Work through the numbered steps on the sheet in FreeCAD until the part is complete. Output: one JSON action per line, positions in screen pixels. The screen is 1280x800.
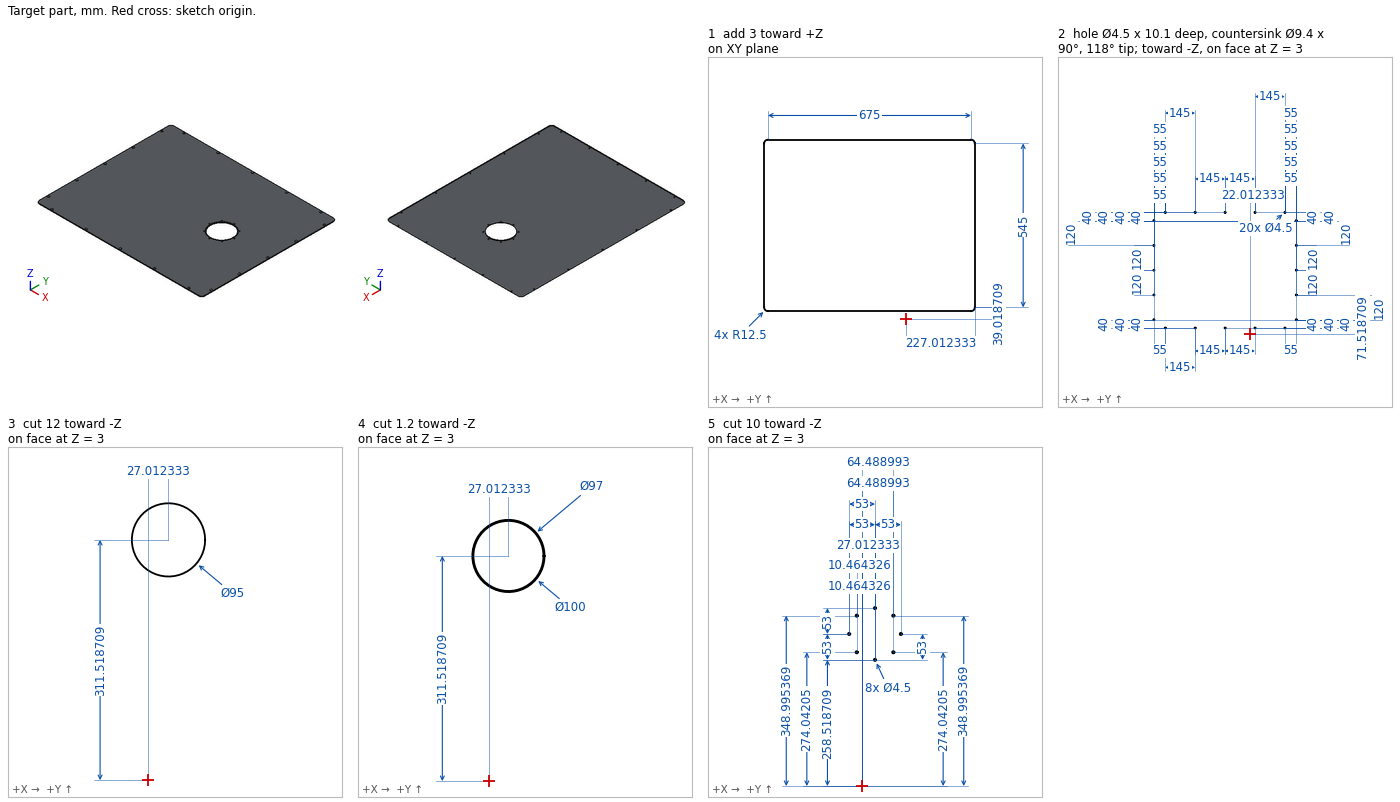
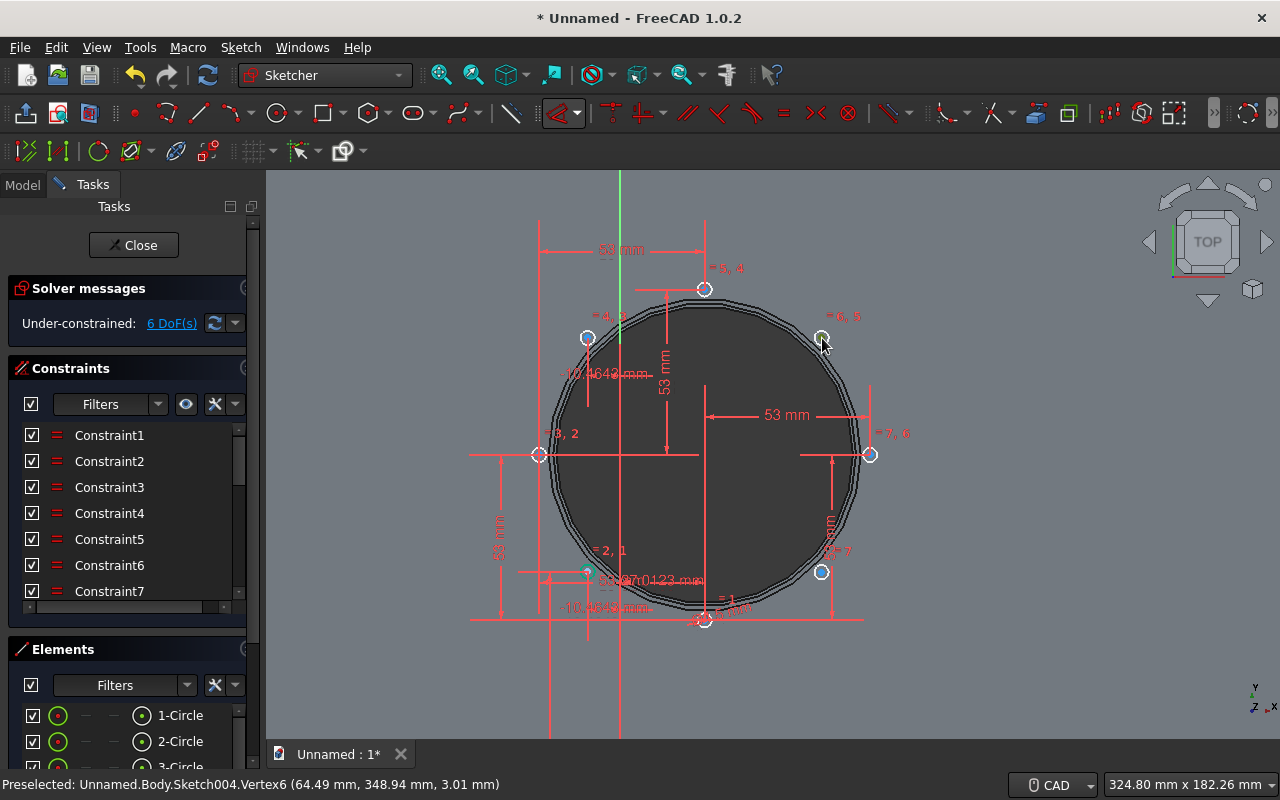
{"action": "key", "text": "l"}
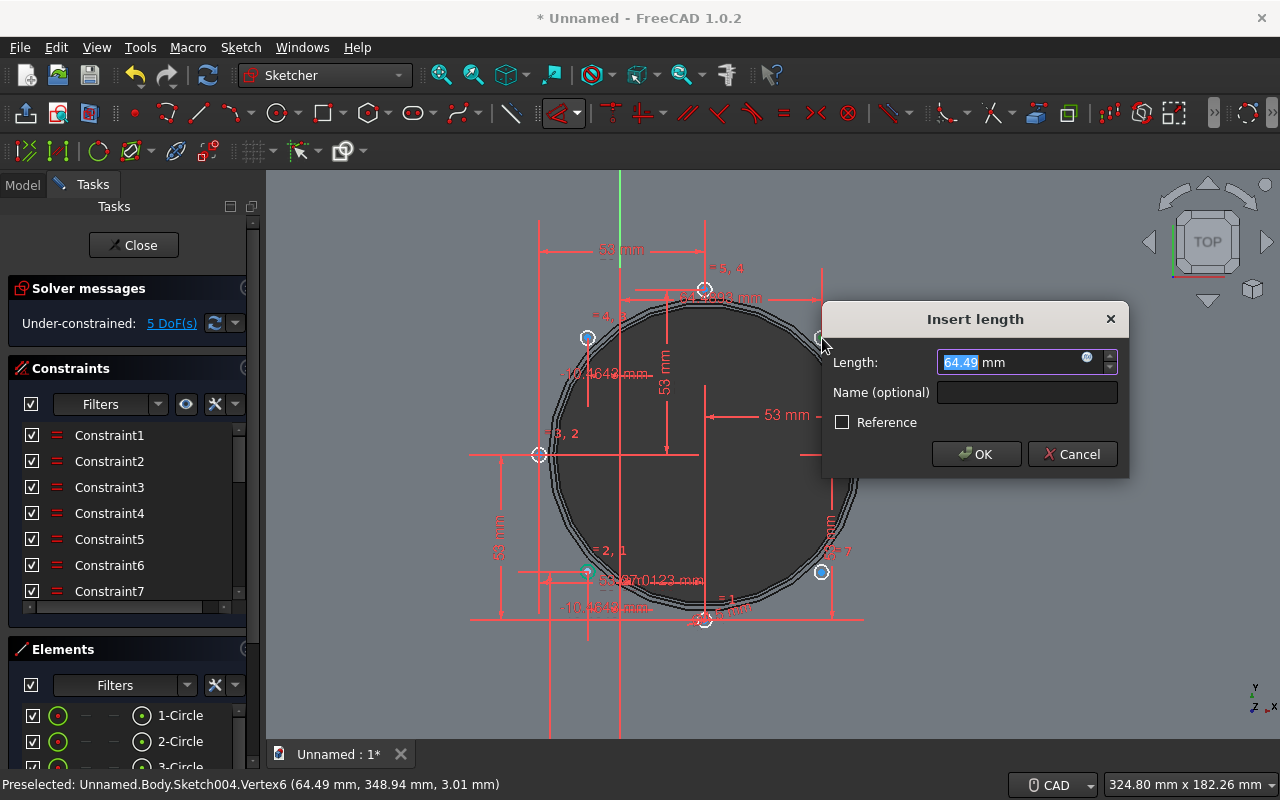
{"action": "type", "text": "64.488993"}
{"action": "key", "text": "Return"}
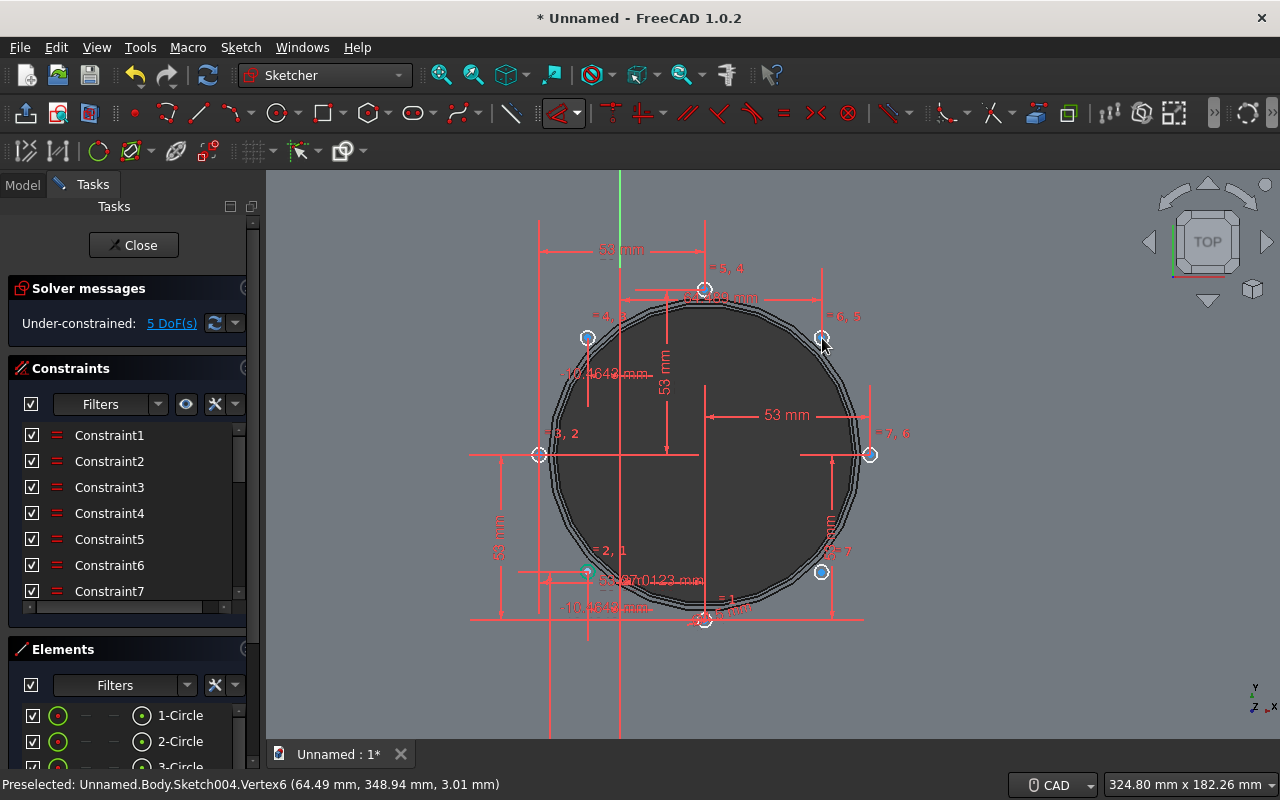
{"action": "left_click", "coordinate": [822, 572]}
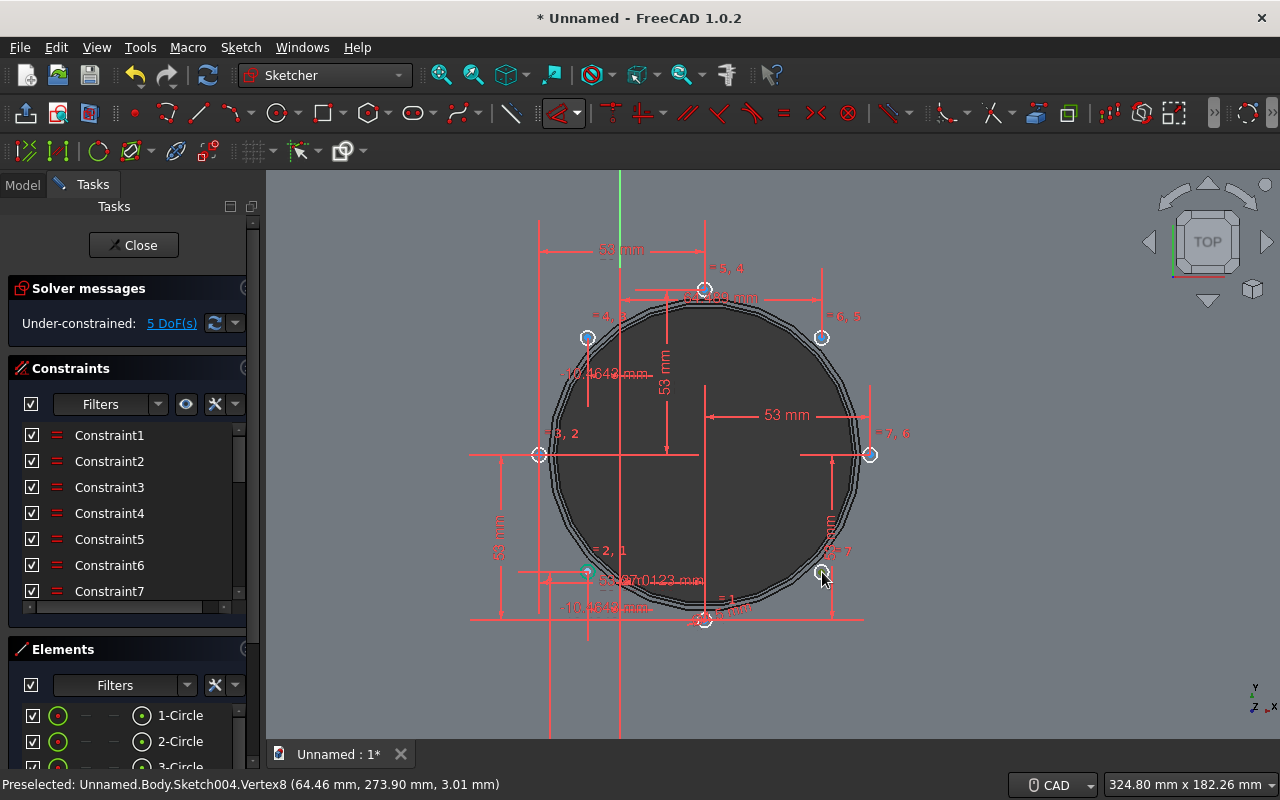
{"action": "key", "text": "l"}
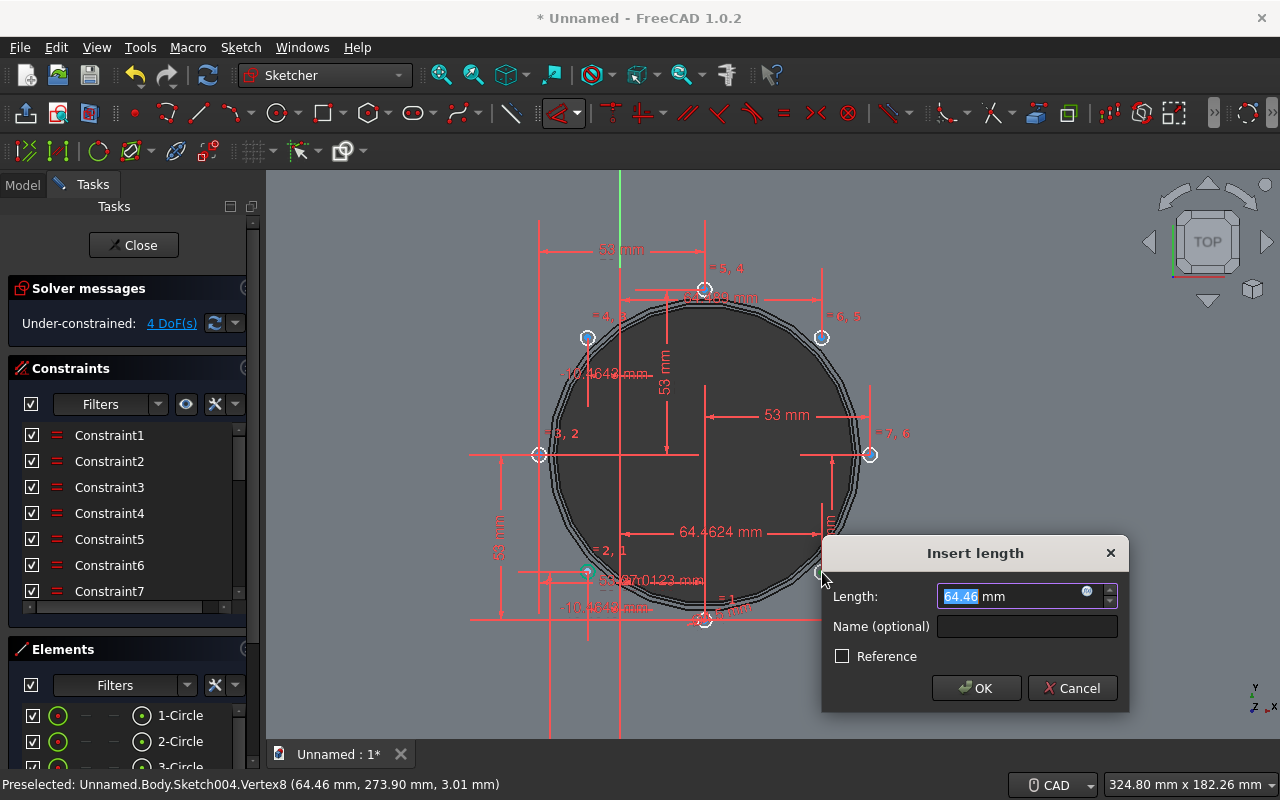
{"action": "type", "text": "64.488993"}
{"action": "key", "text": "Return"}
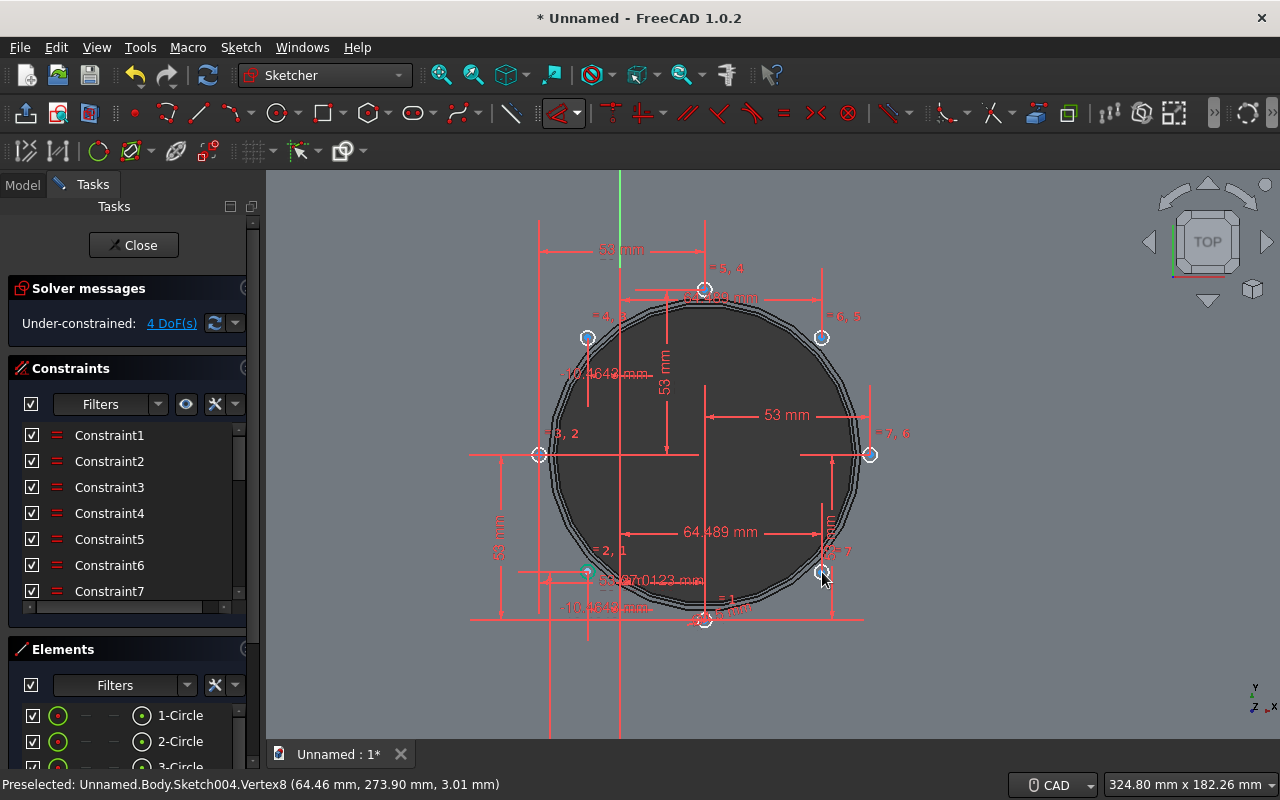
{"action": "left_click", "coordinate": [822, 572]}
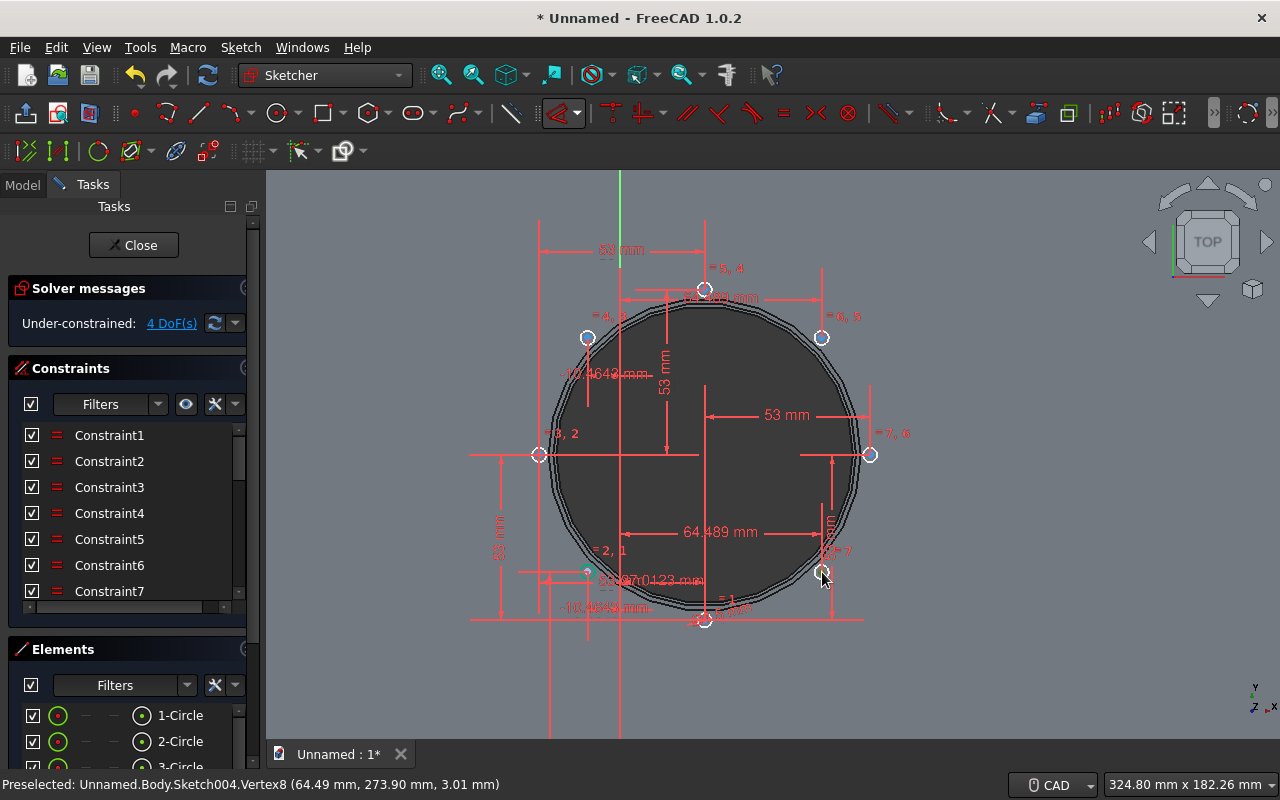
{"action": "left_click", "coordinate": [580, 114]}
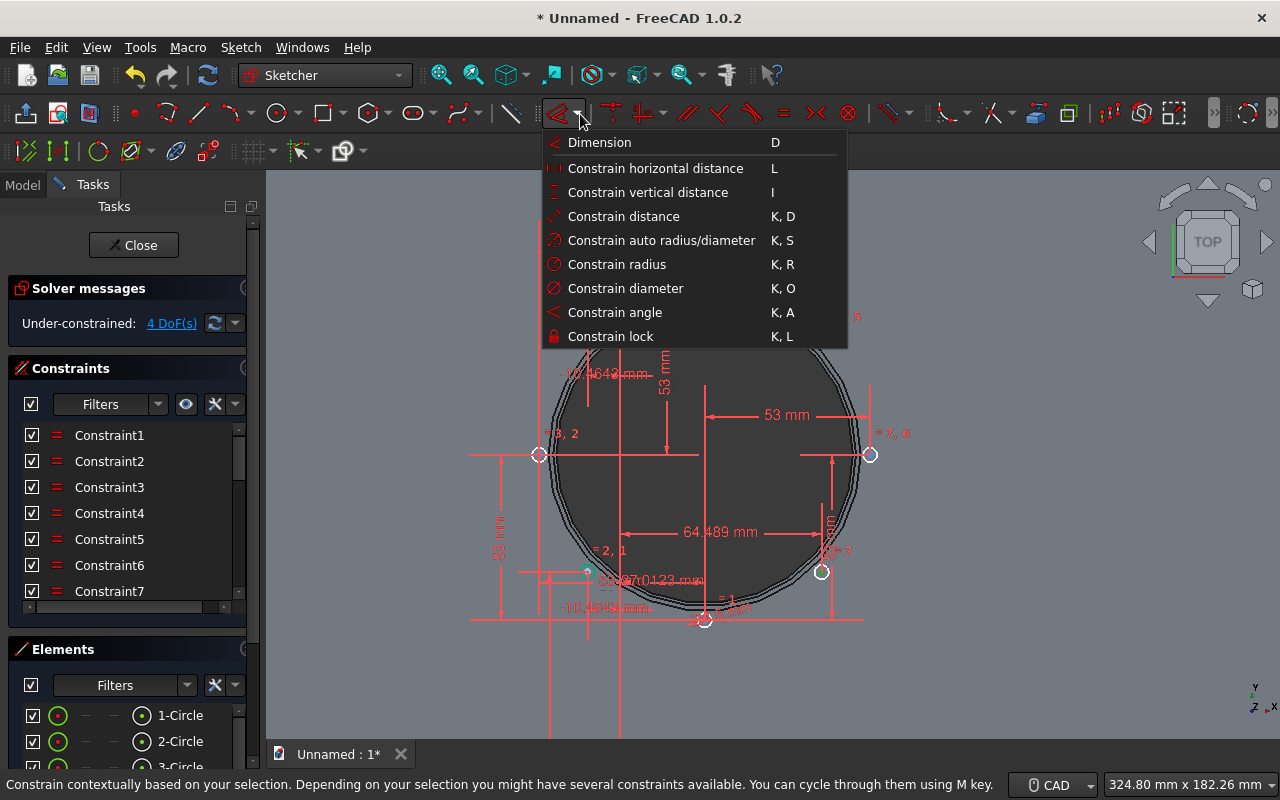
{"action": "left_click", "coordinate": [695, 192]}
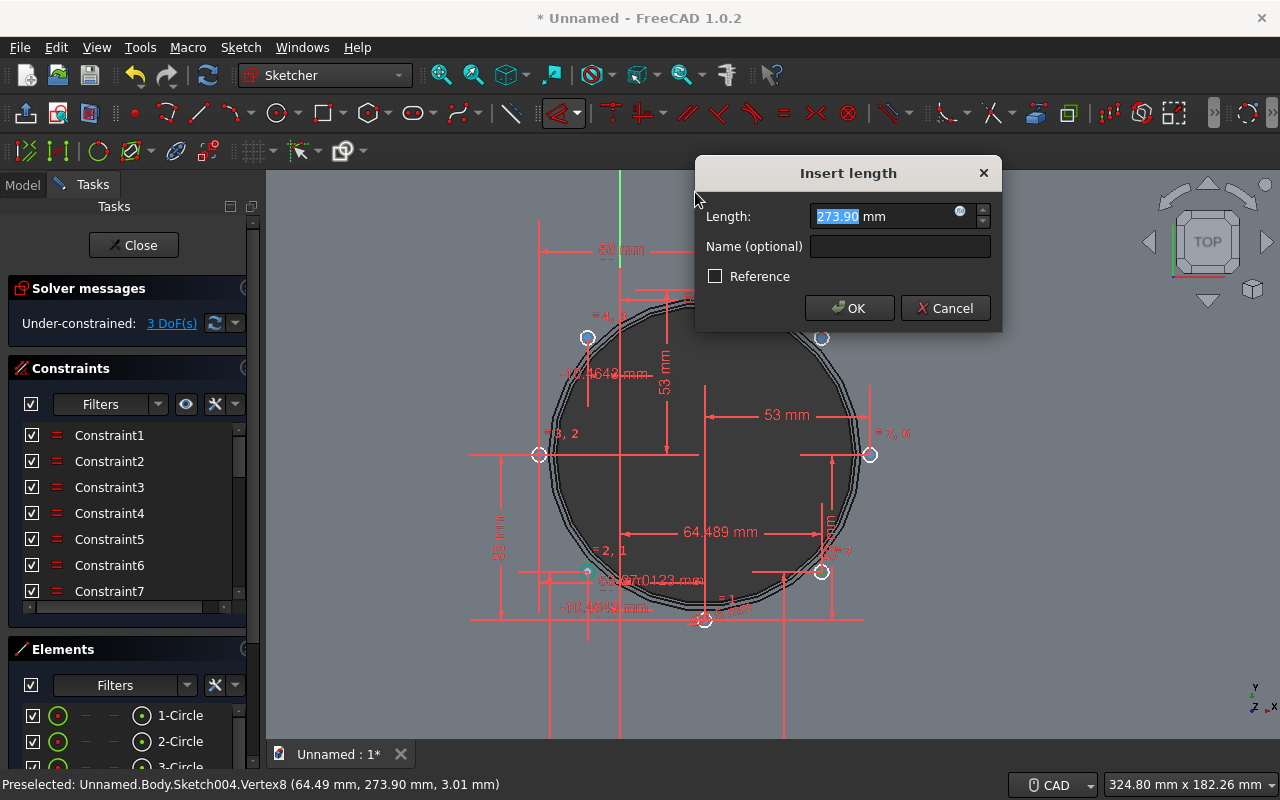
{"action": "type", "text": "274.04205"}
{"action": "key", "text": "Return"}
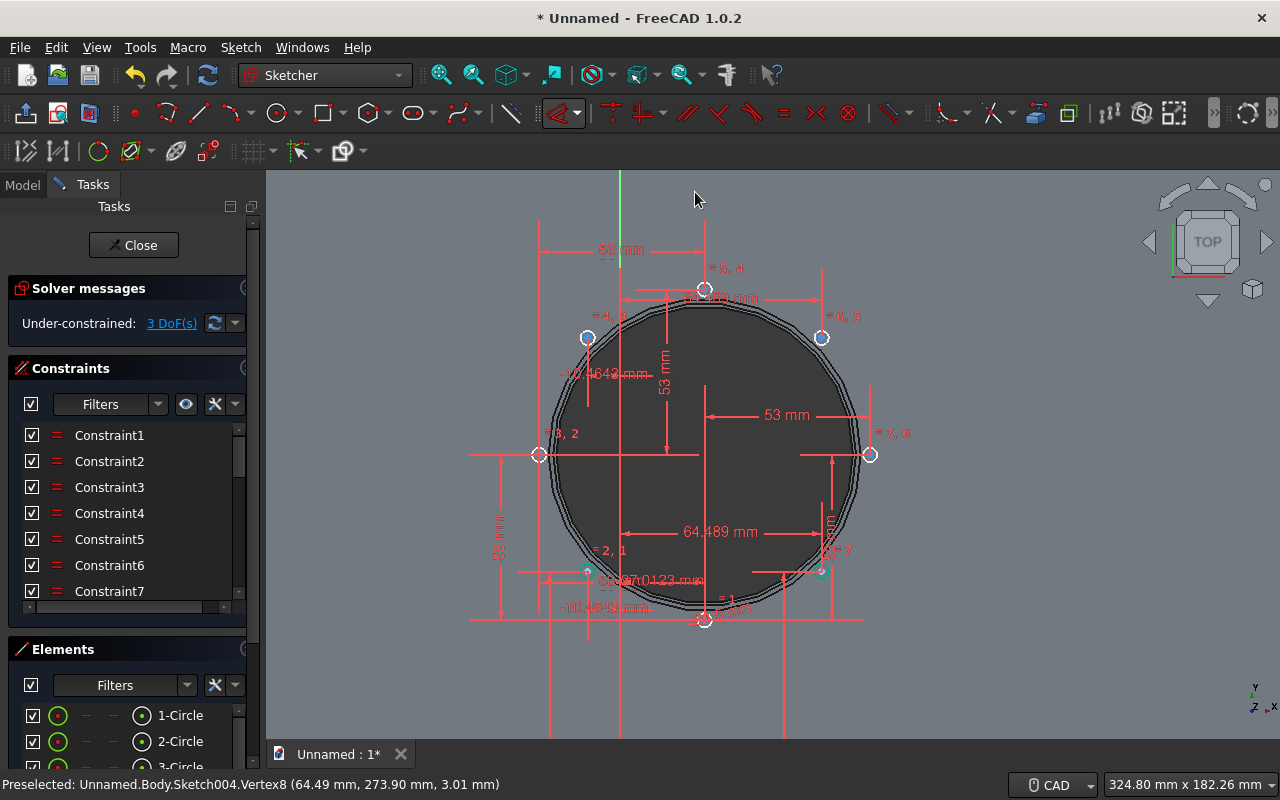
{"action": "left_click", "coordinate": [705, 620]}